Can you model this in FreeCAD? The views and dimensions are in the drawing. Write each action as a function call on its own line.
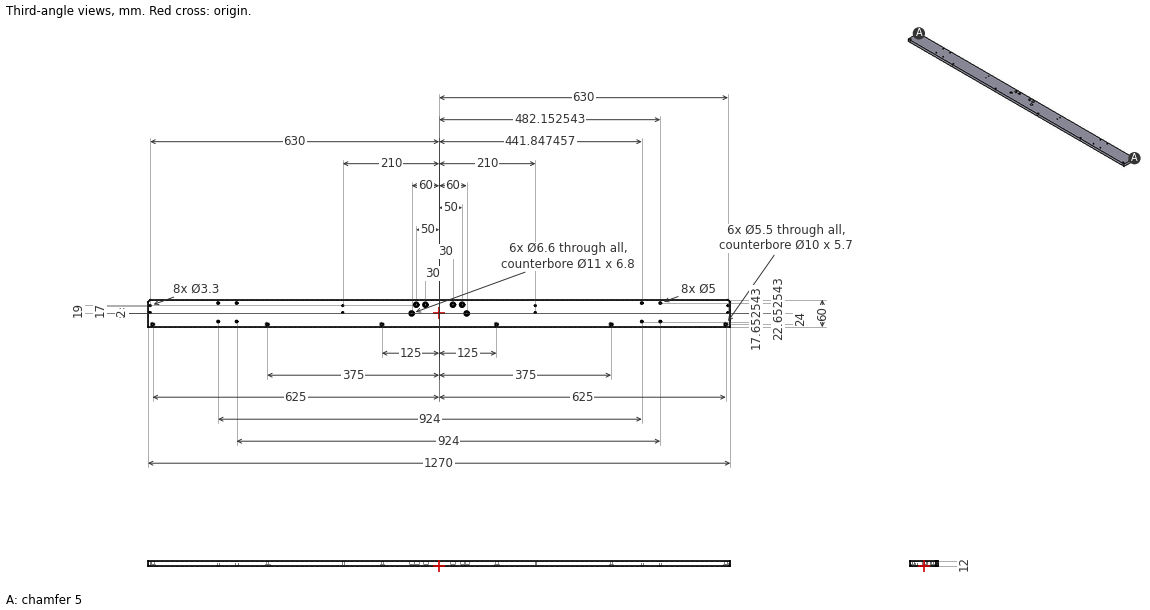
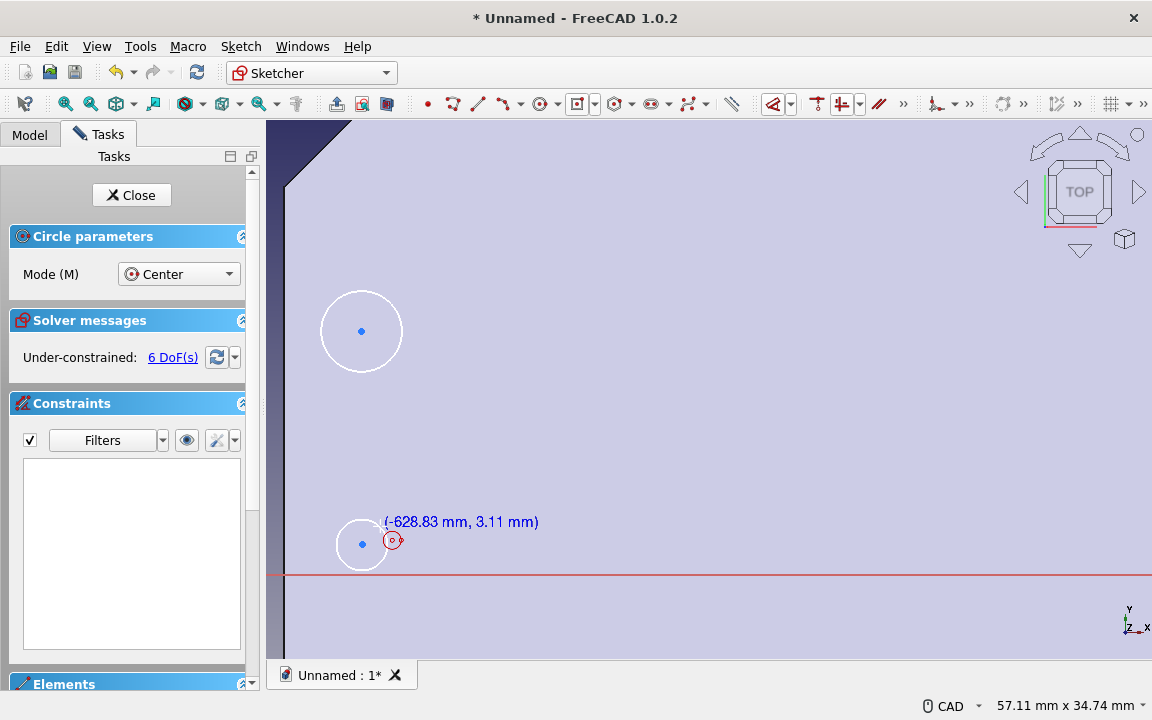
scroll(374, 388, down, 18)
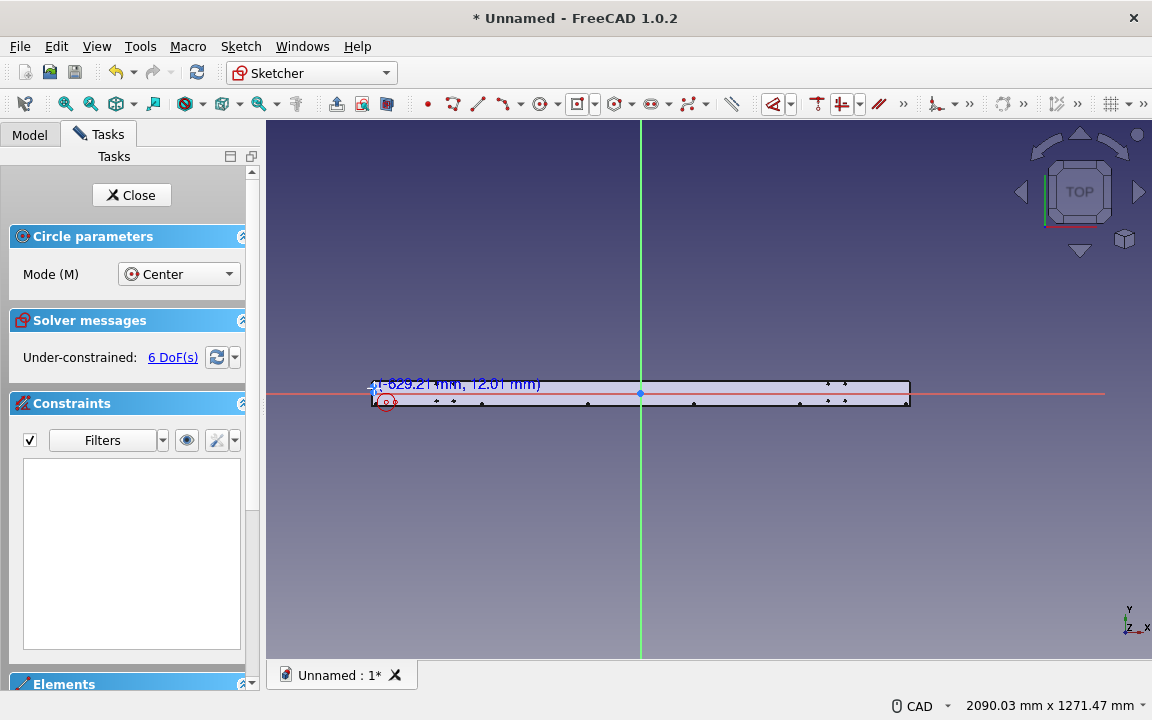
scroll(908, 393, up, 18)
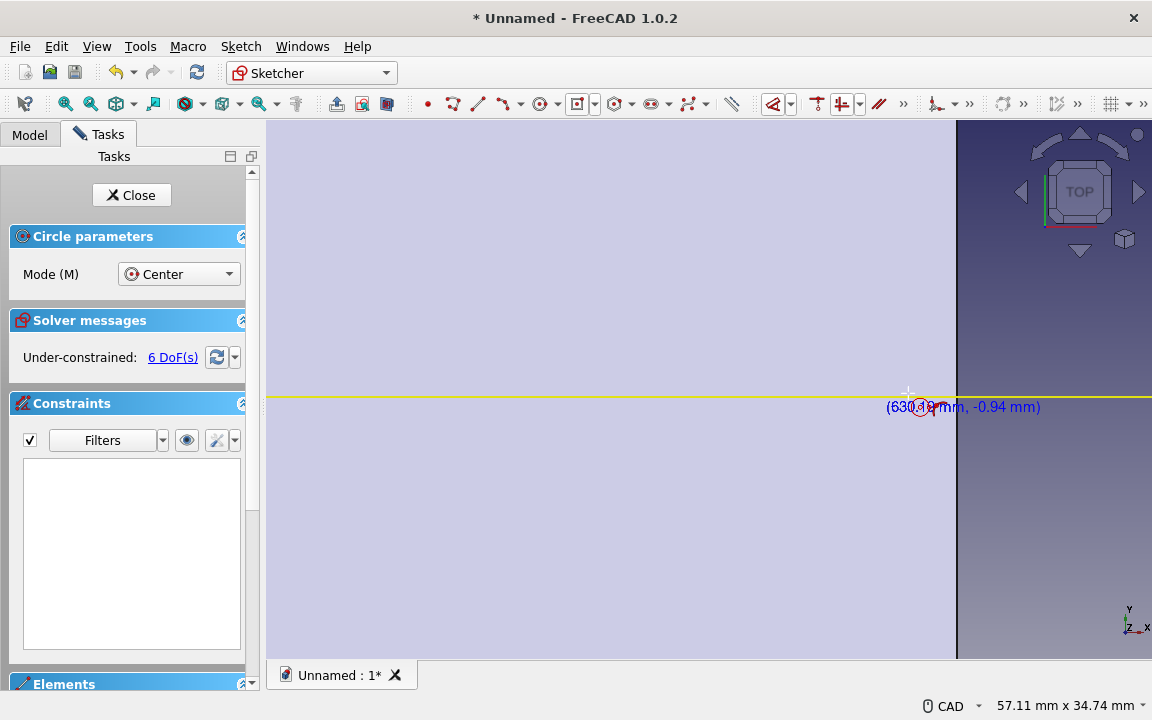
click(879, 366)
click(897, 348)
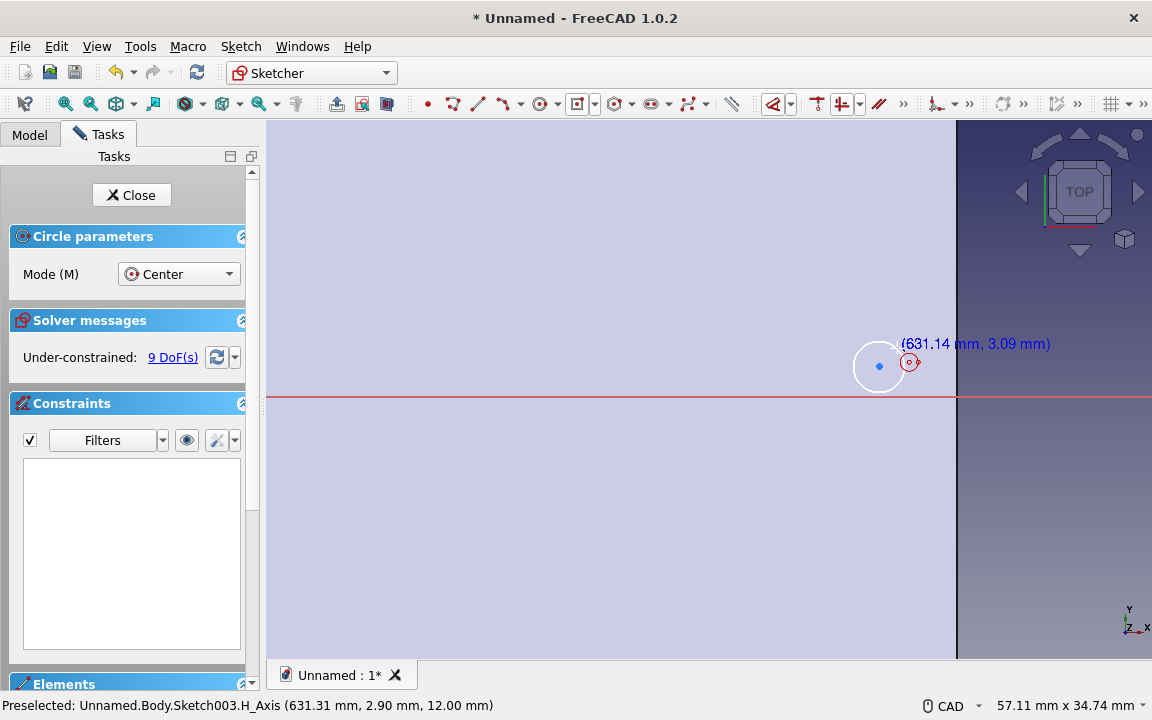
scroll(908, 393, down, 18)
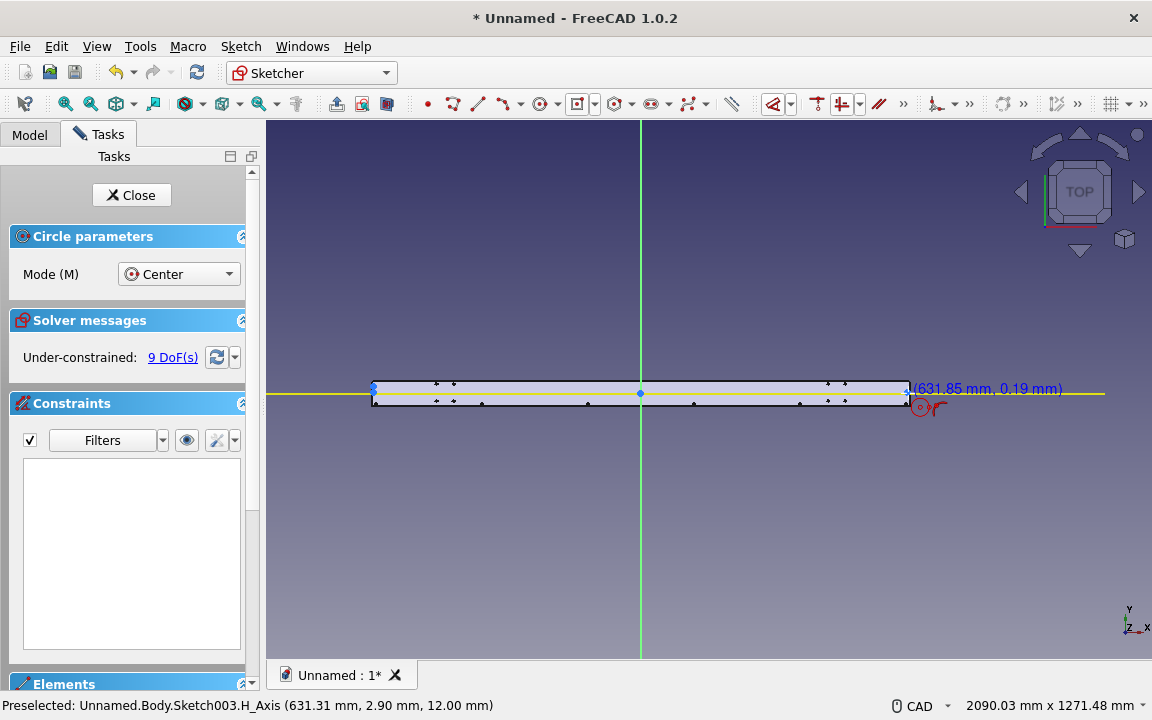
scroll(908, 386, up, 18)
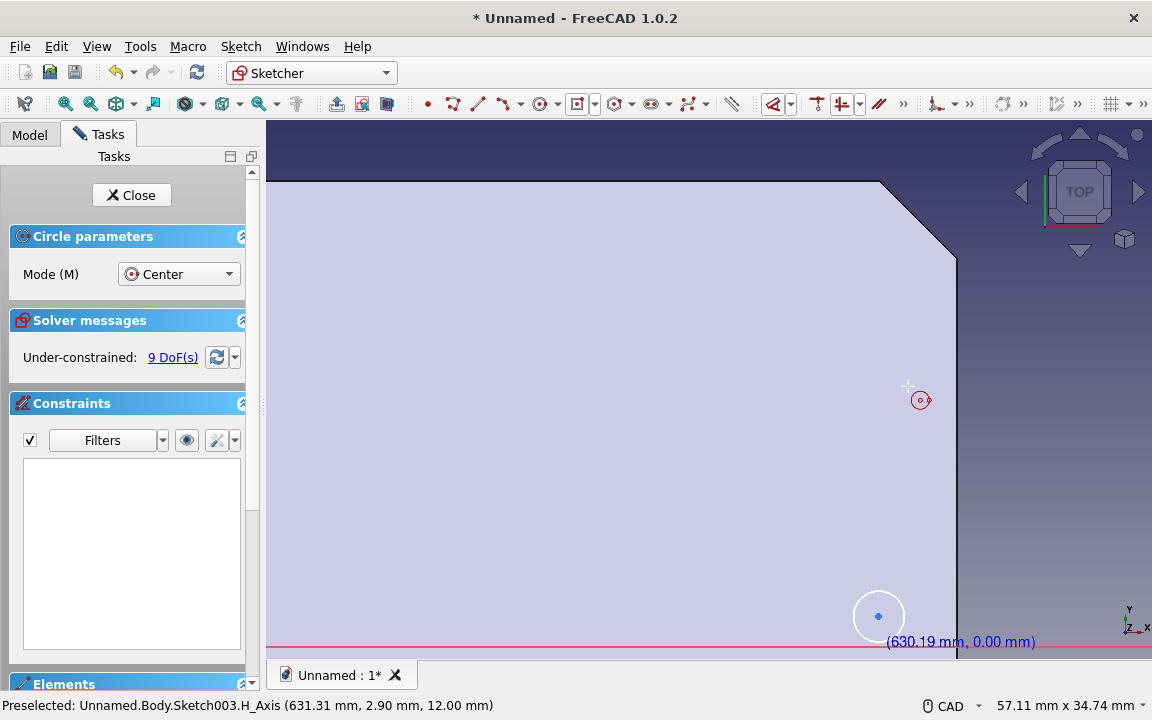
scroll(908, 386, down, 18)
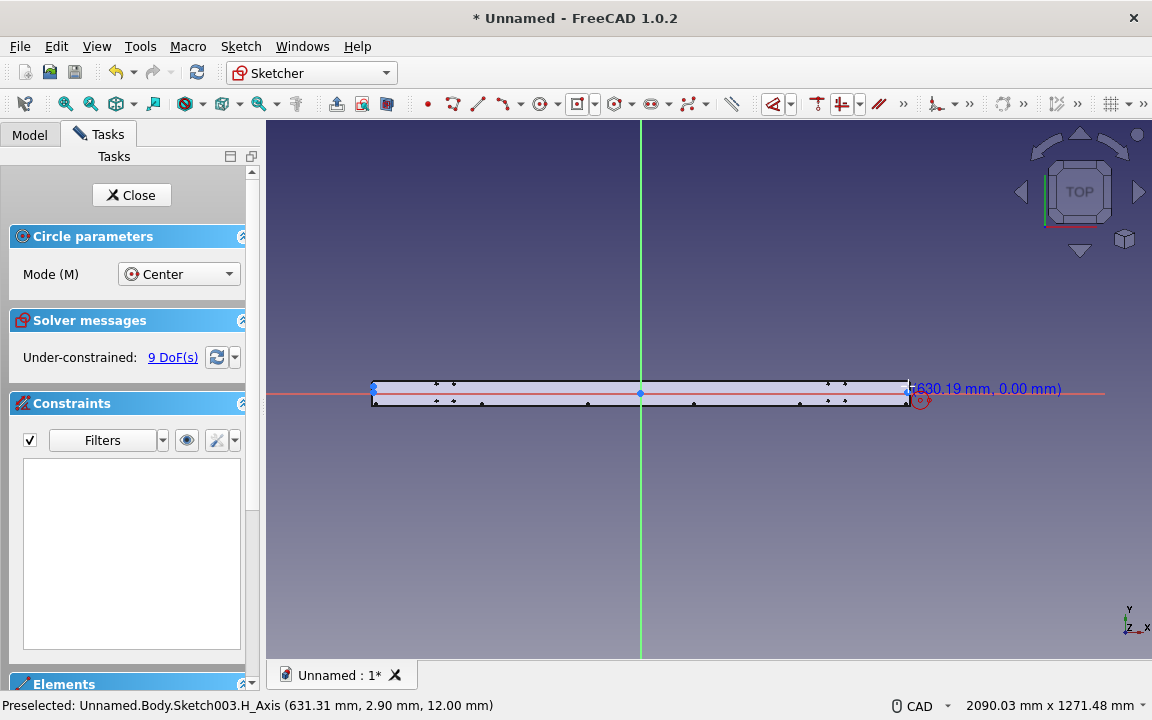
scroll(908, 386, up, 6)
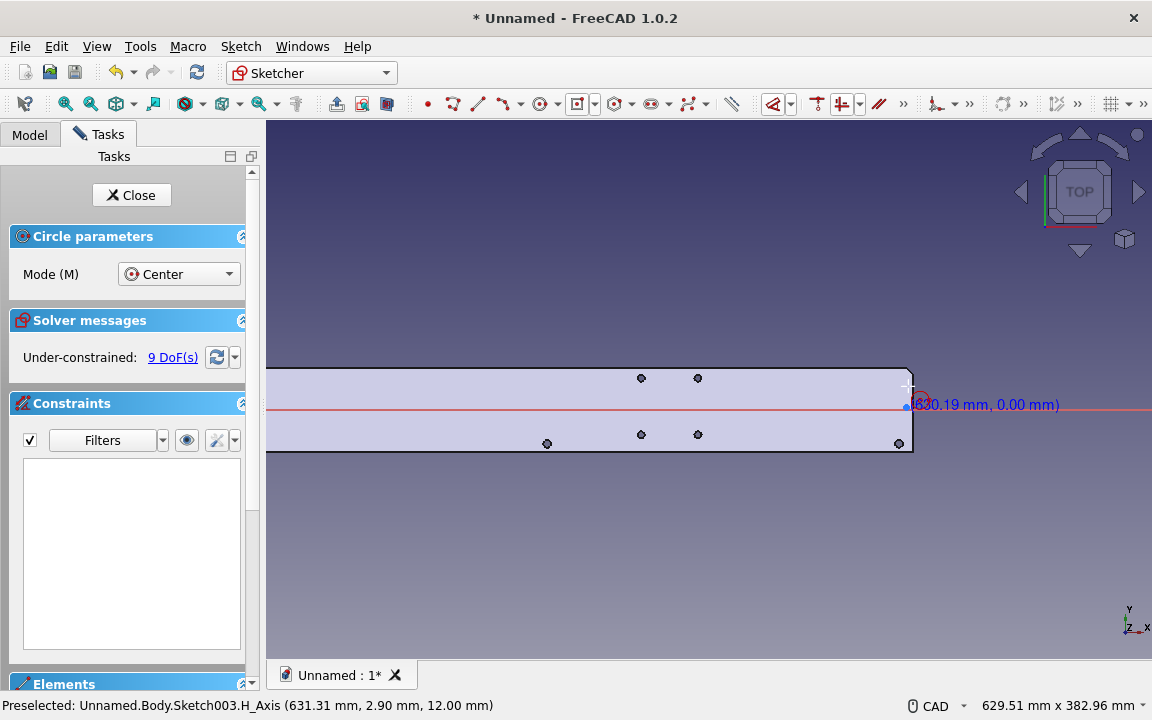
click(906, 386)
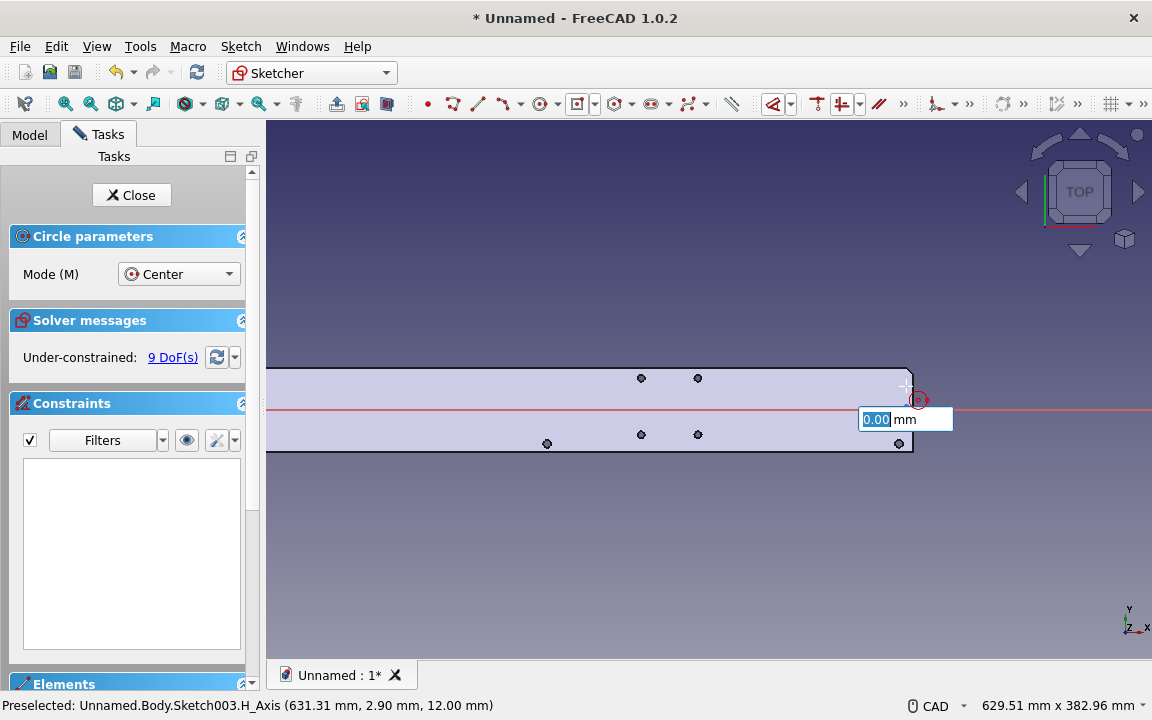
scroll(908, 385, up, 10)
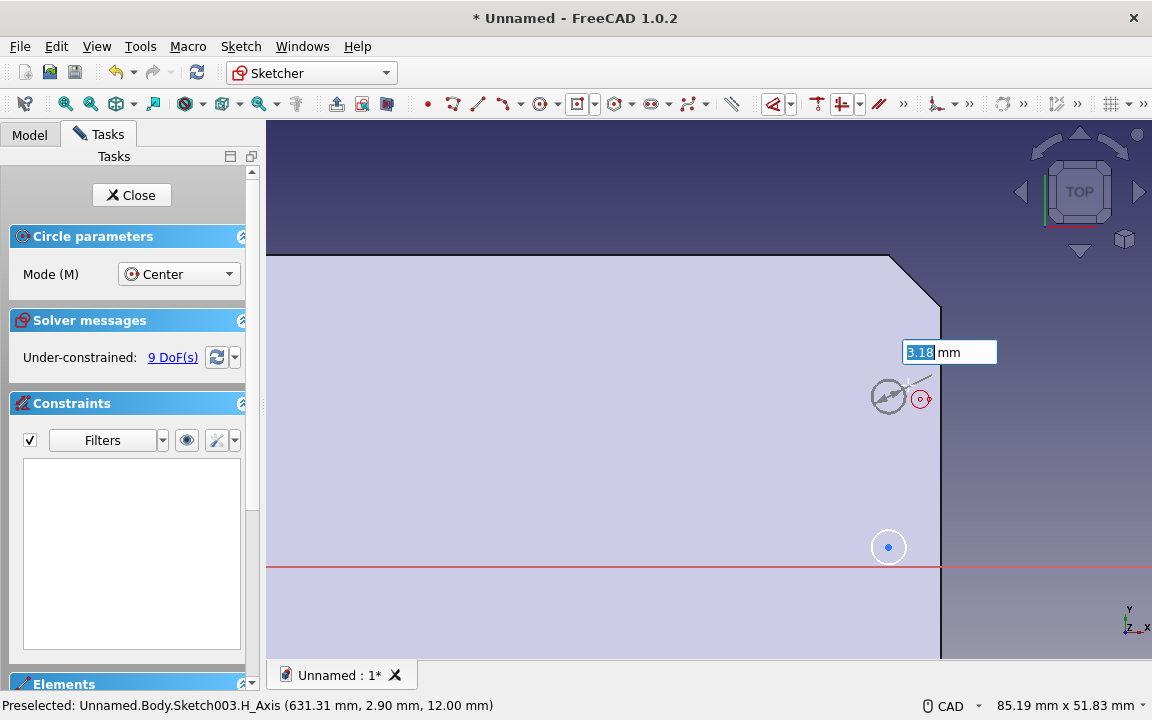
click(901, 378)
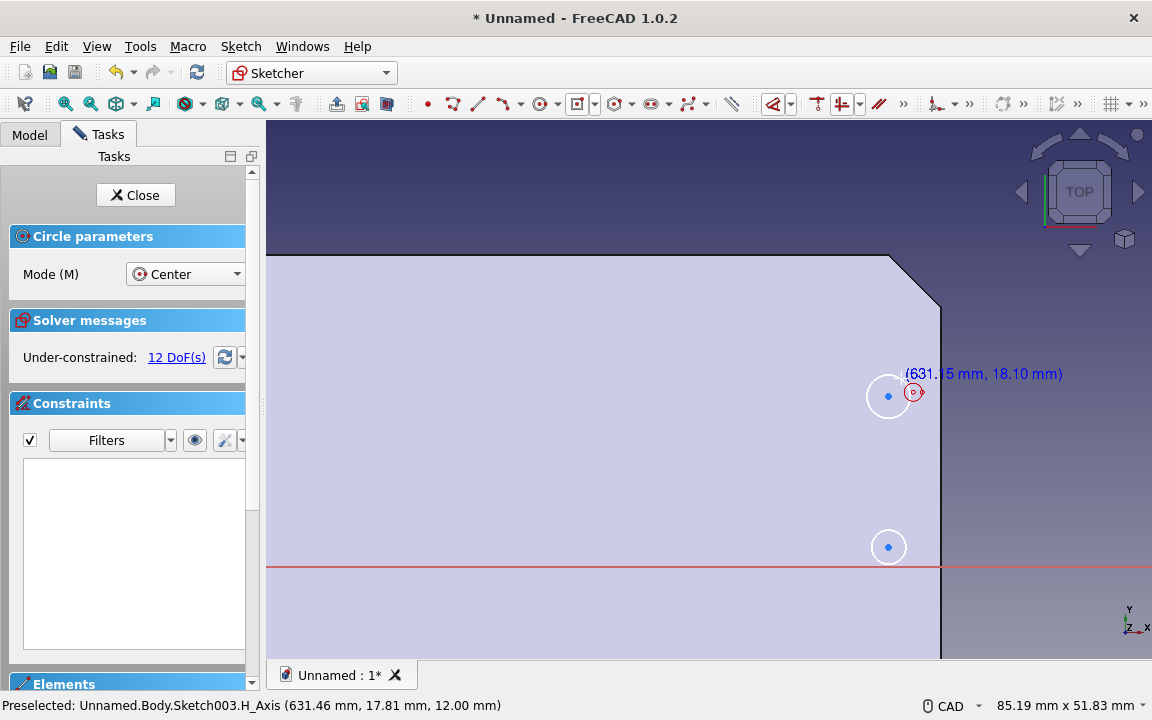
scroll(908, 386, down, 16)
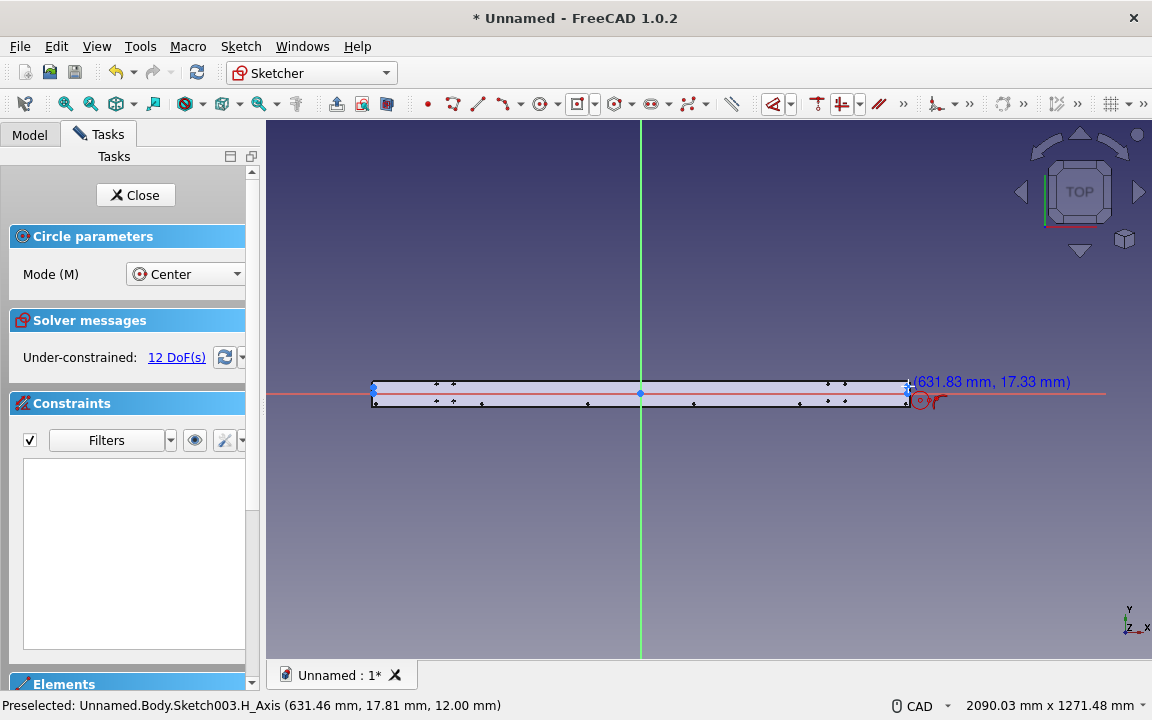
scroll(552, 387, up, 18)